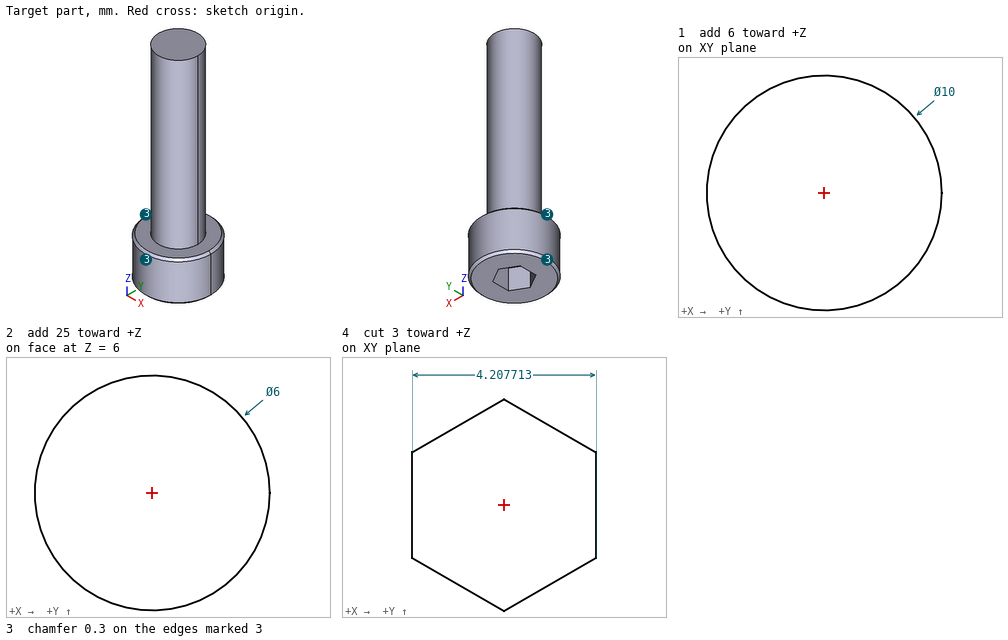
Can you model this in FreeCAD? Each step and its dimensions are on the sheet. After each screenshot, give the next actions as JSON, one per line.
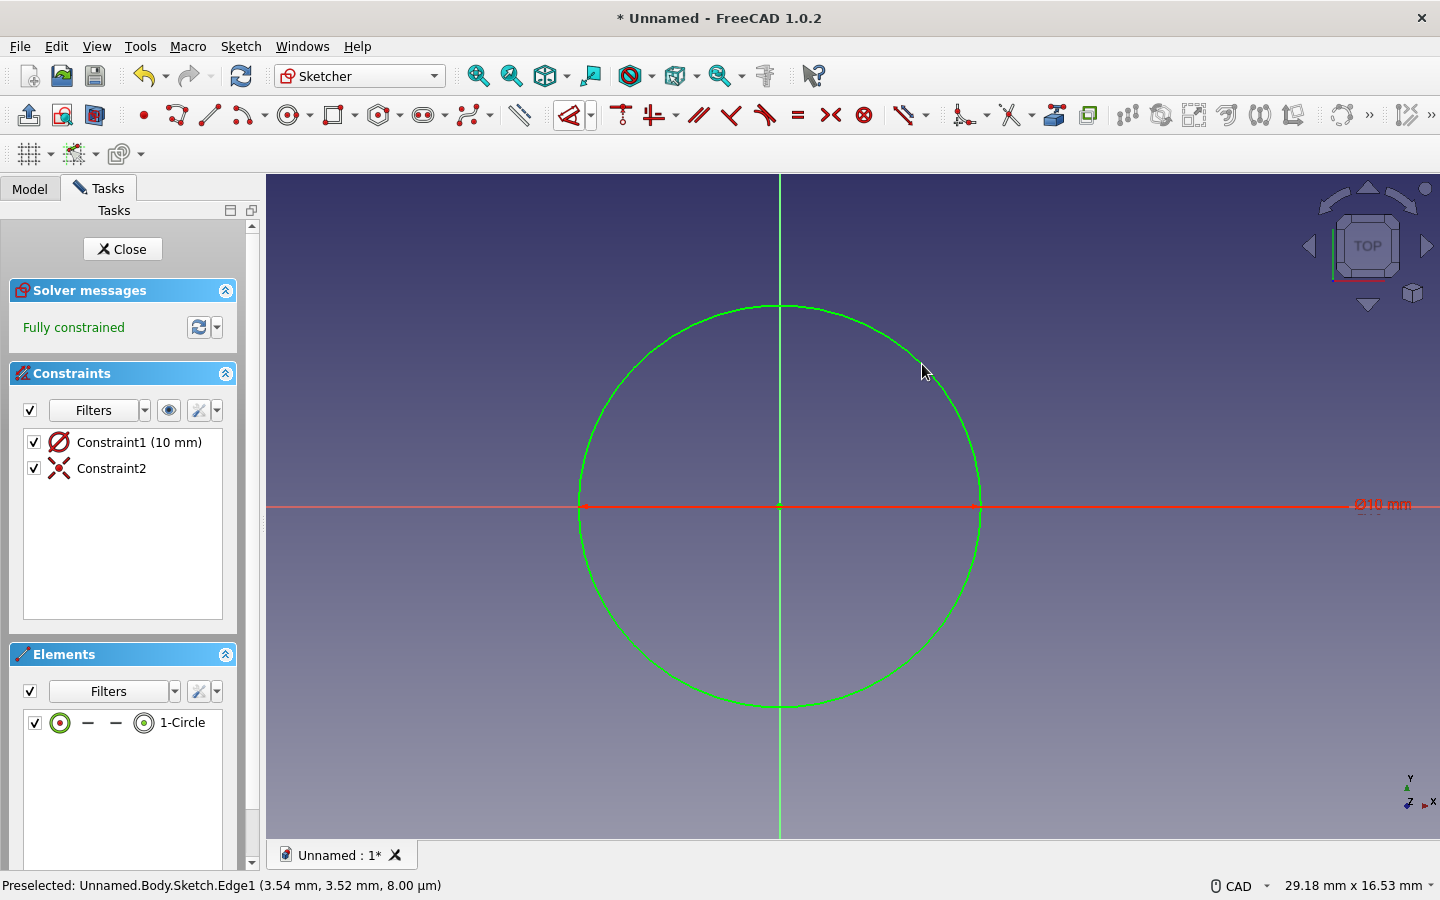
{"action": "left_click", "coordinate": [123, 249]}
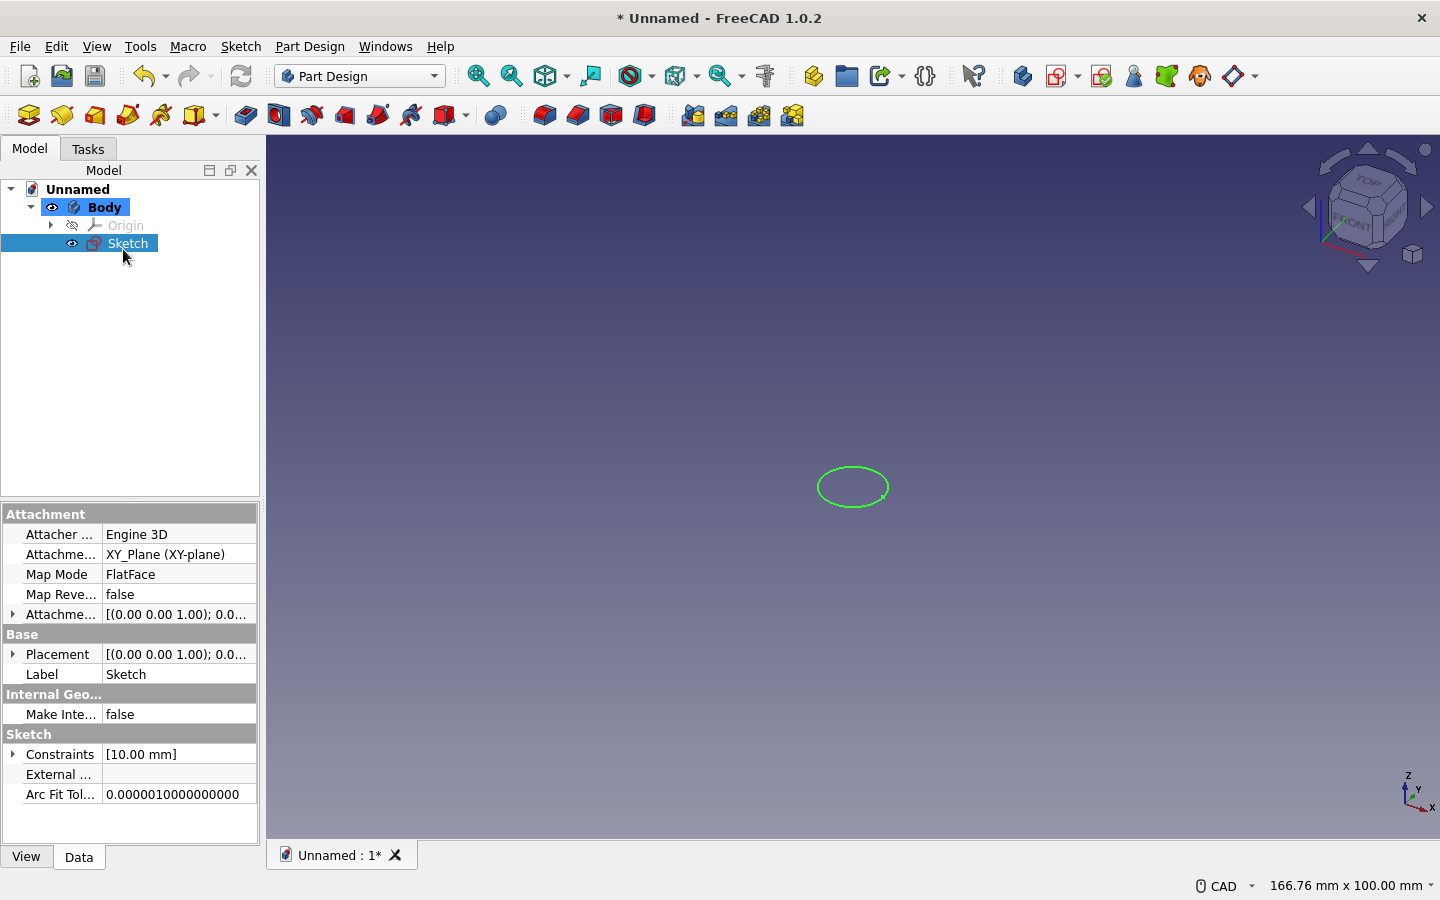
{"action": "left_click", "coordinate": [29, 116]}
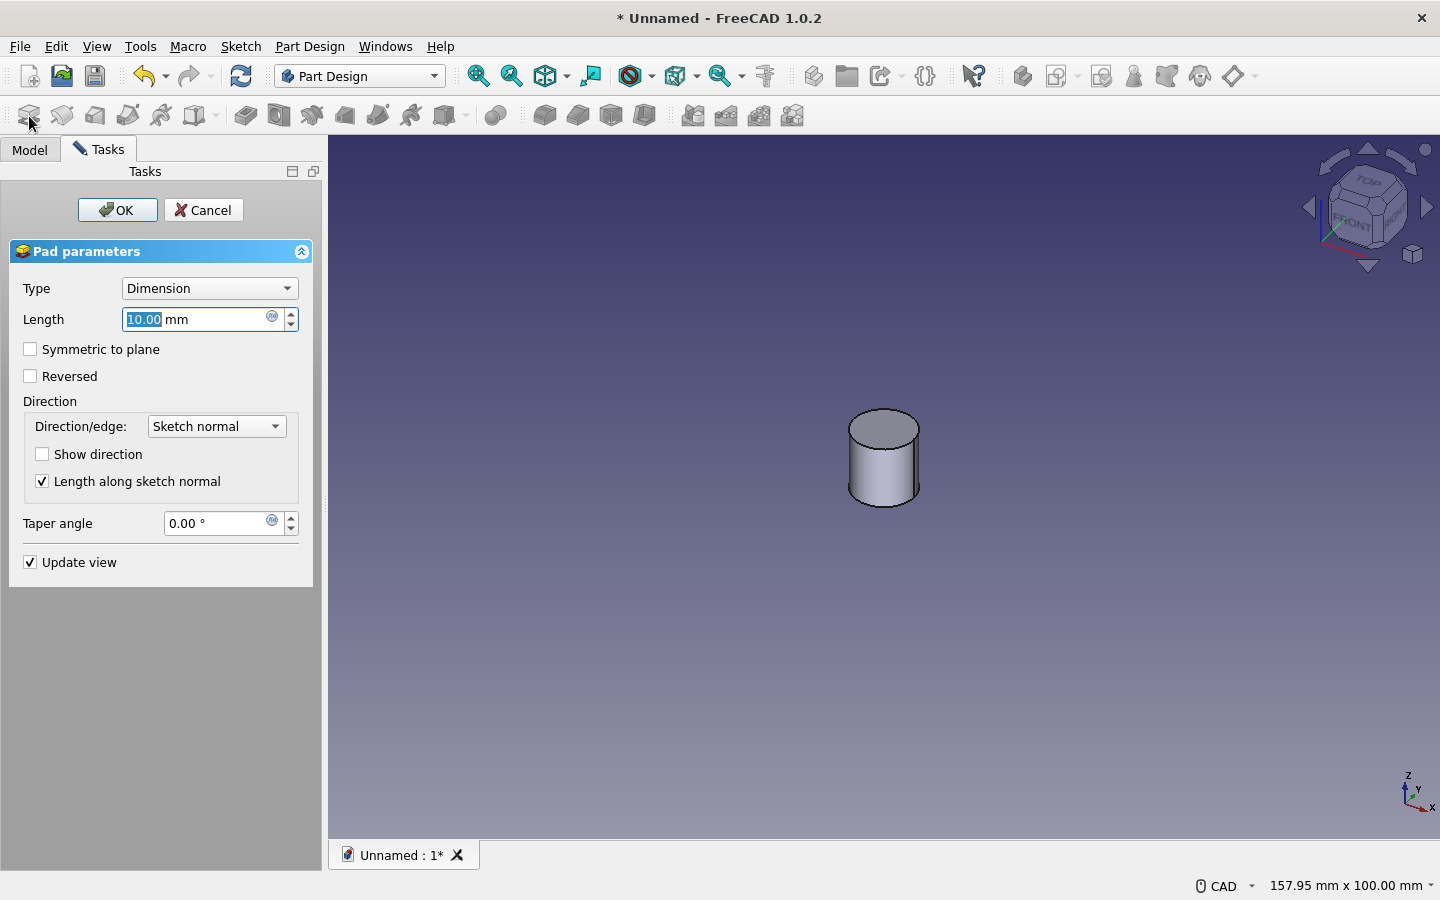
{"action": "type", "text": "6"}
{"action": "key", "text": "Tab"}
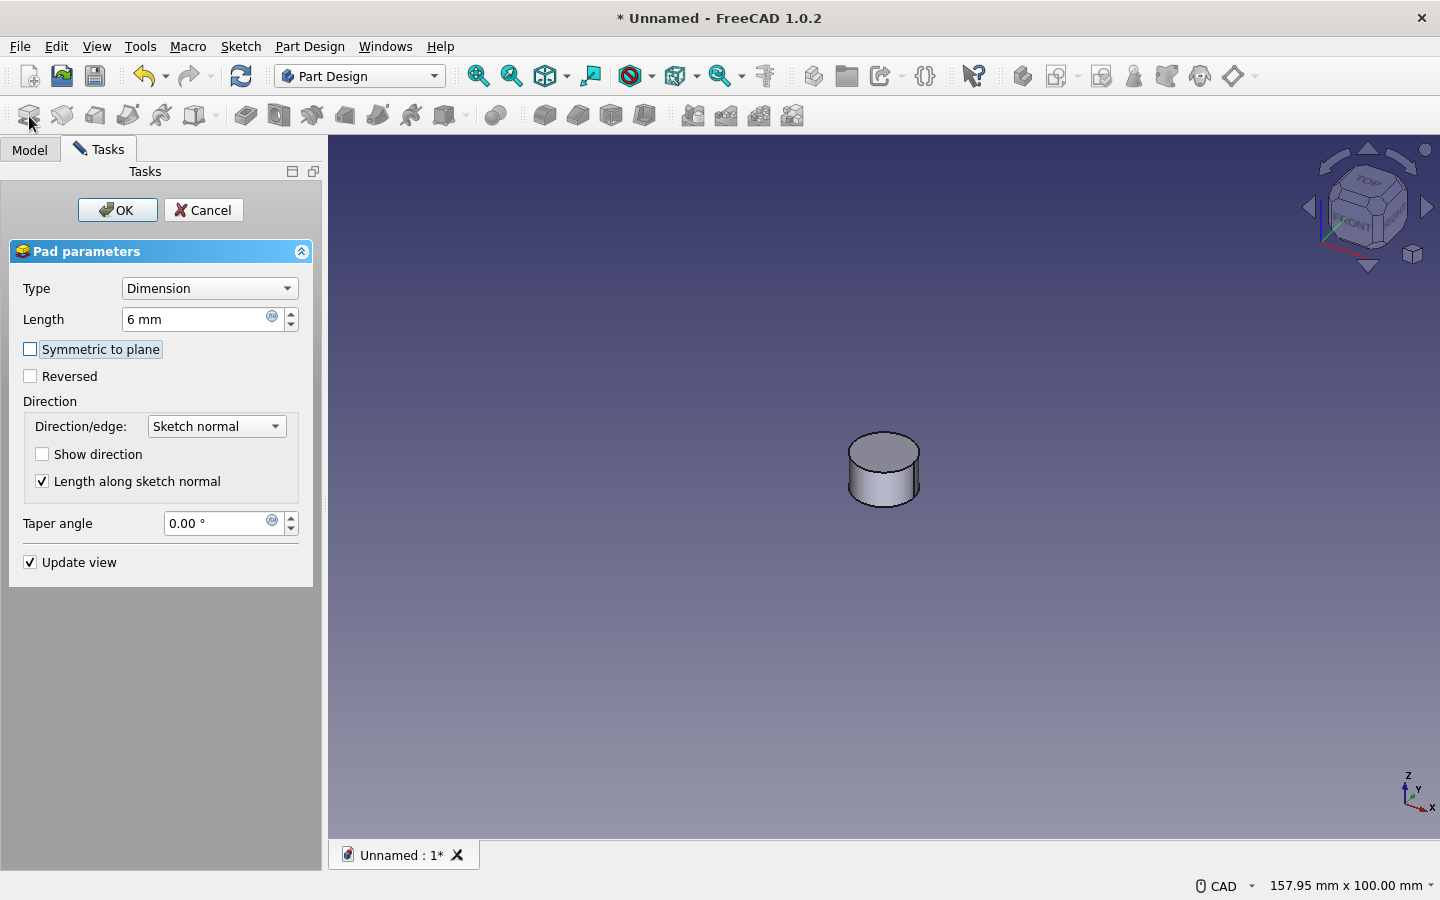
{"action": "left_click", "coordinate": [118, 210]}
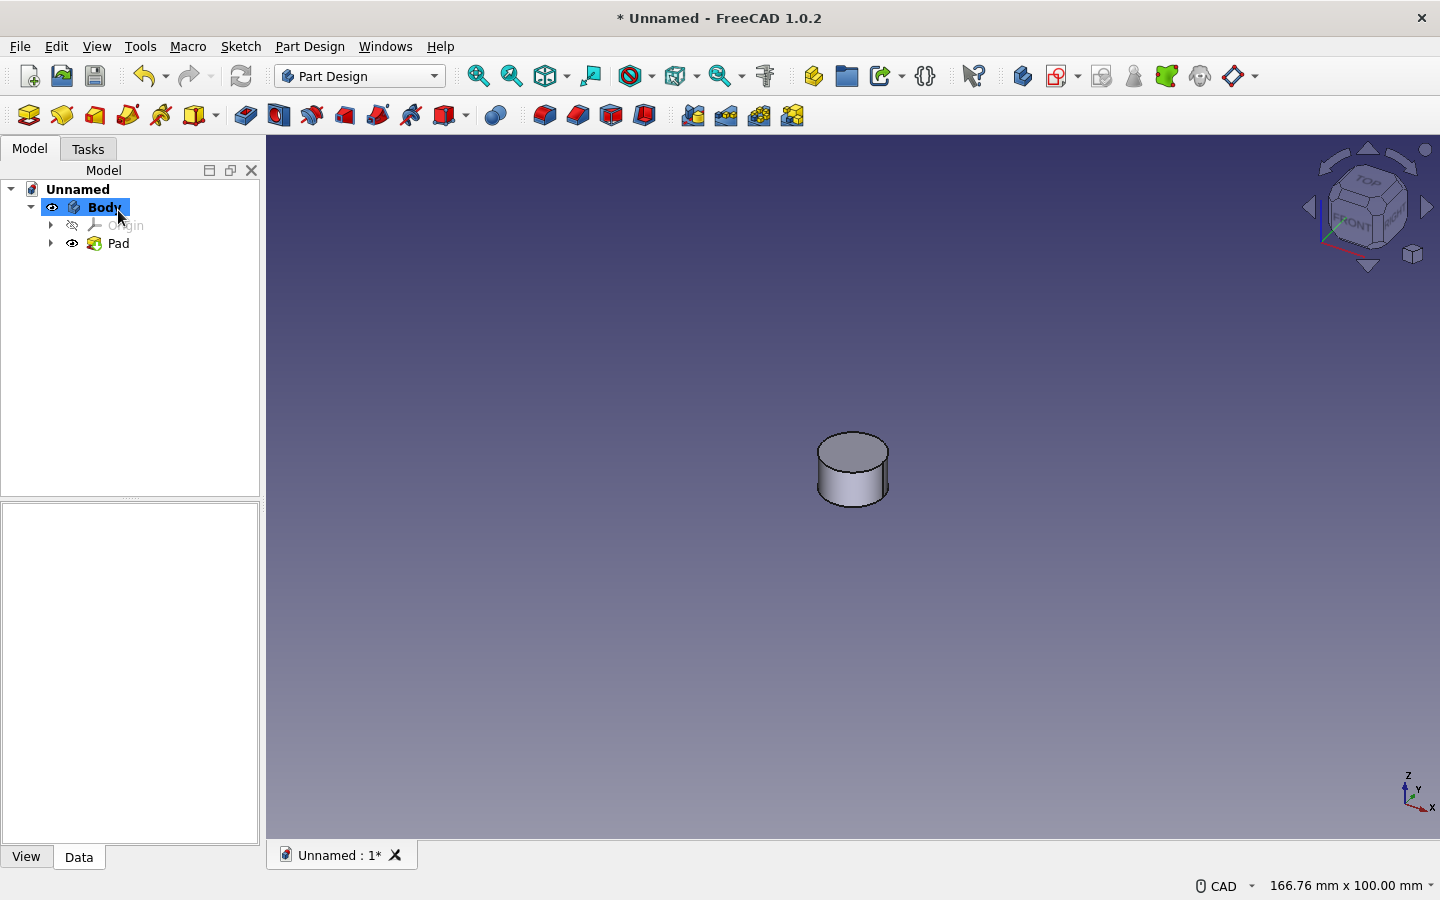
{"action": "key", "text": "v f"}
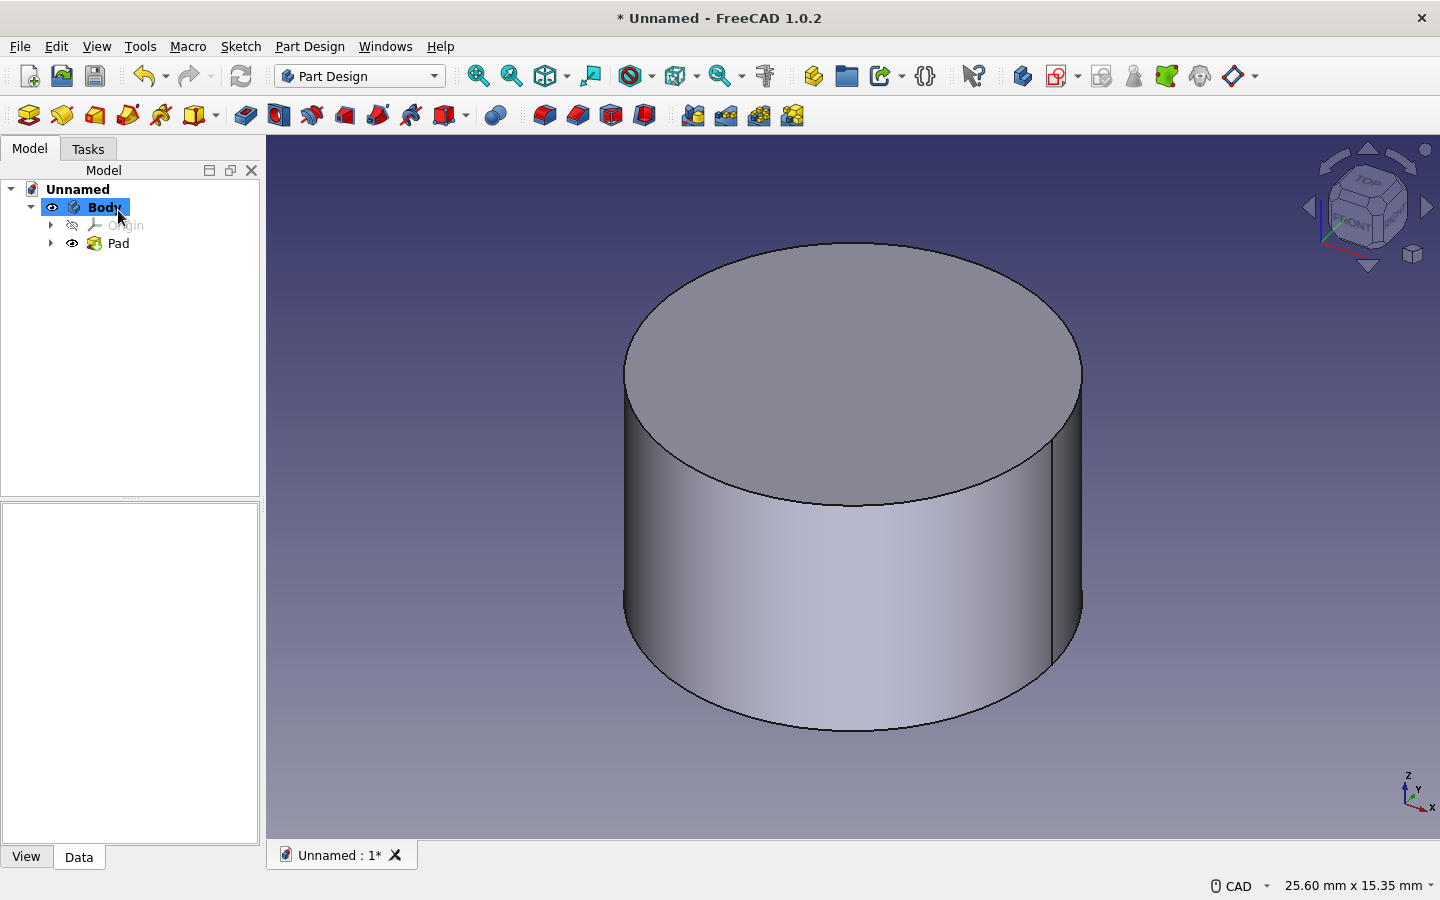
{"action": "left_click", "coordinate": [853, 373]}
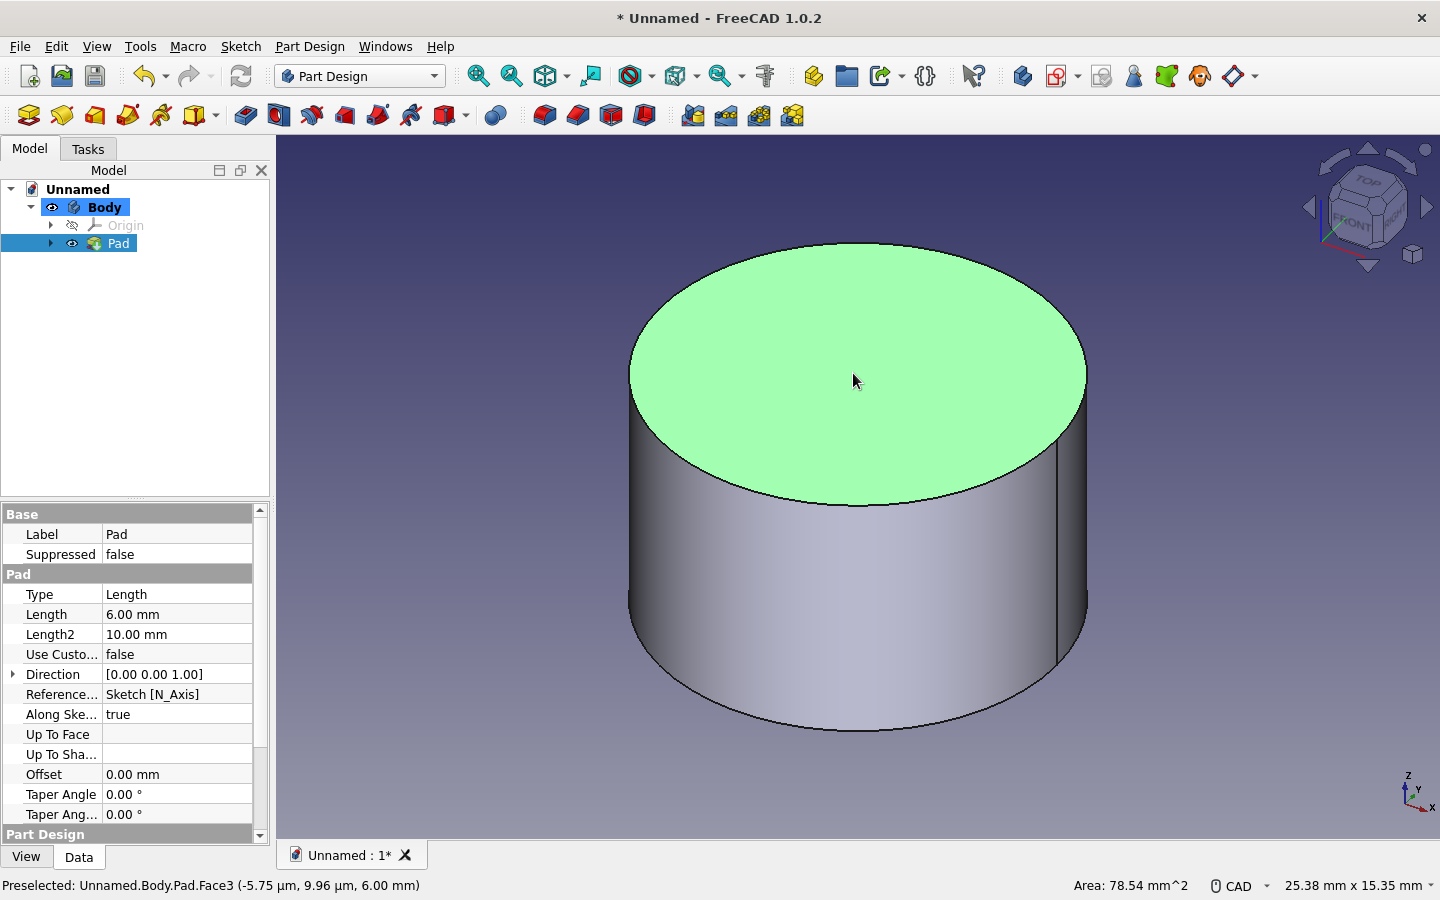
{"action": "left_click", "coordinate": [1056, 76]}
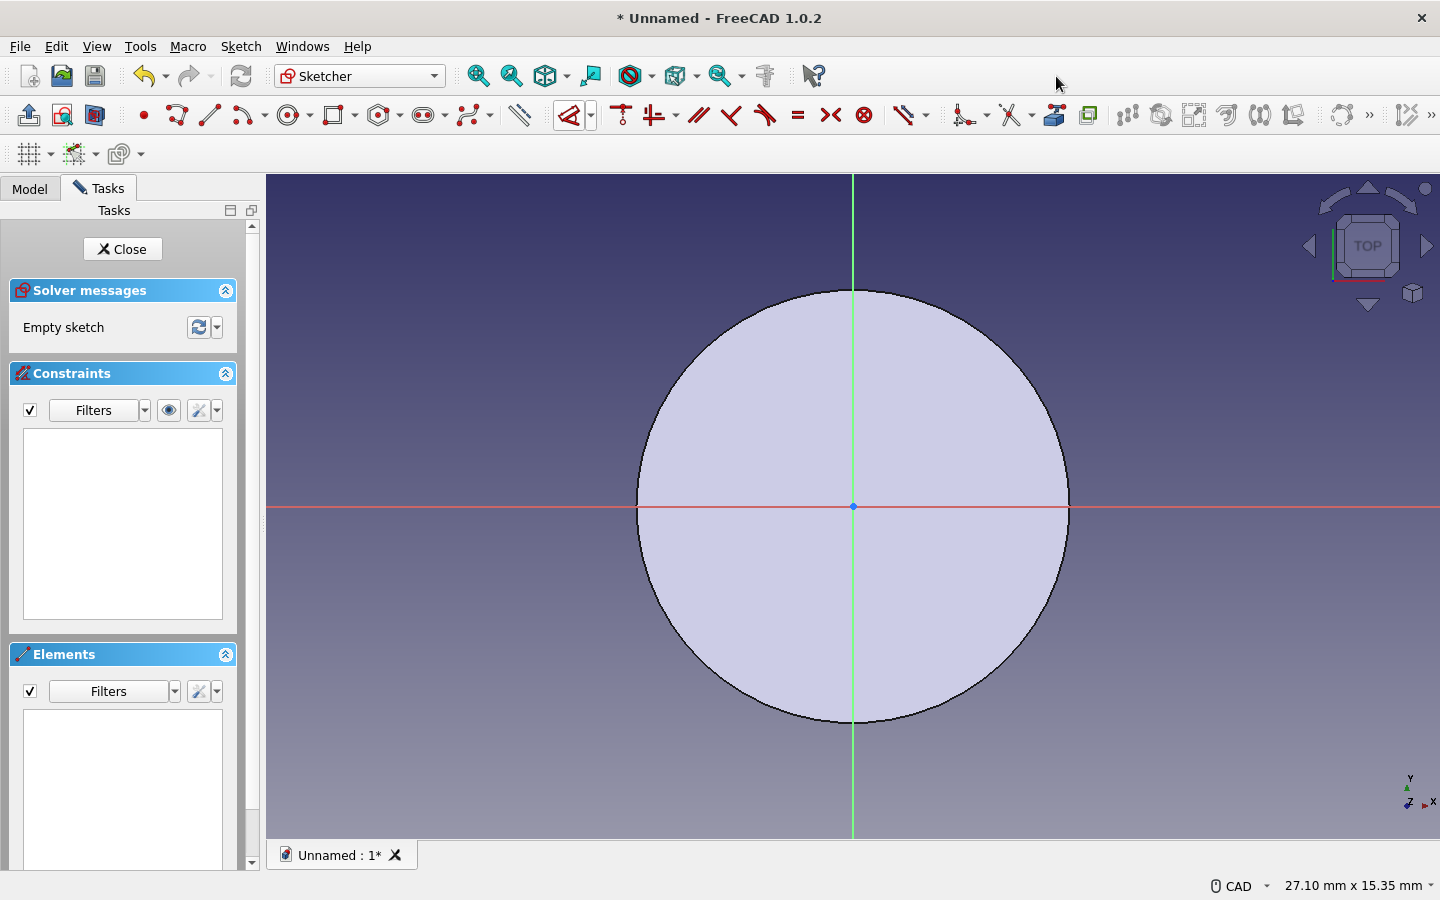
{"action": "scroll", "coordinate": [936, 507], "scroll_direction": "up", "scroll_amount": 3}